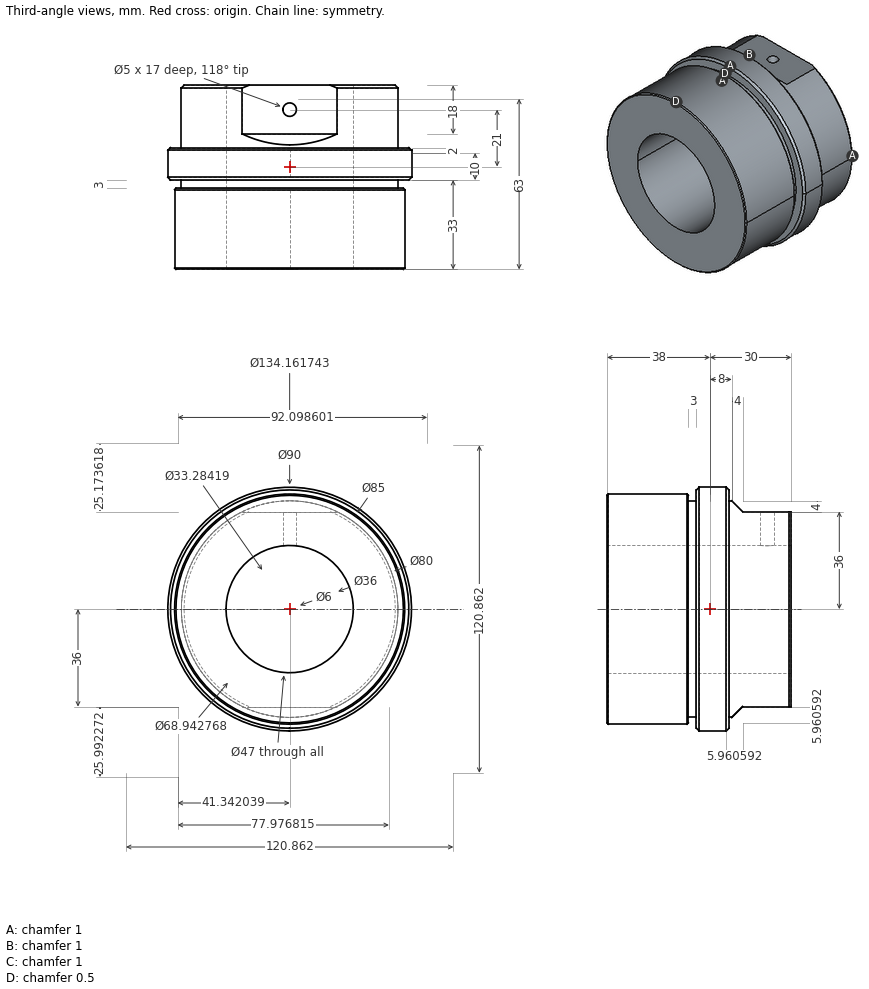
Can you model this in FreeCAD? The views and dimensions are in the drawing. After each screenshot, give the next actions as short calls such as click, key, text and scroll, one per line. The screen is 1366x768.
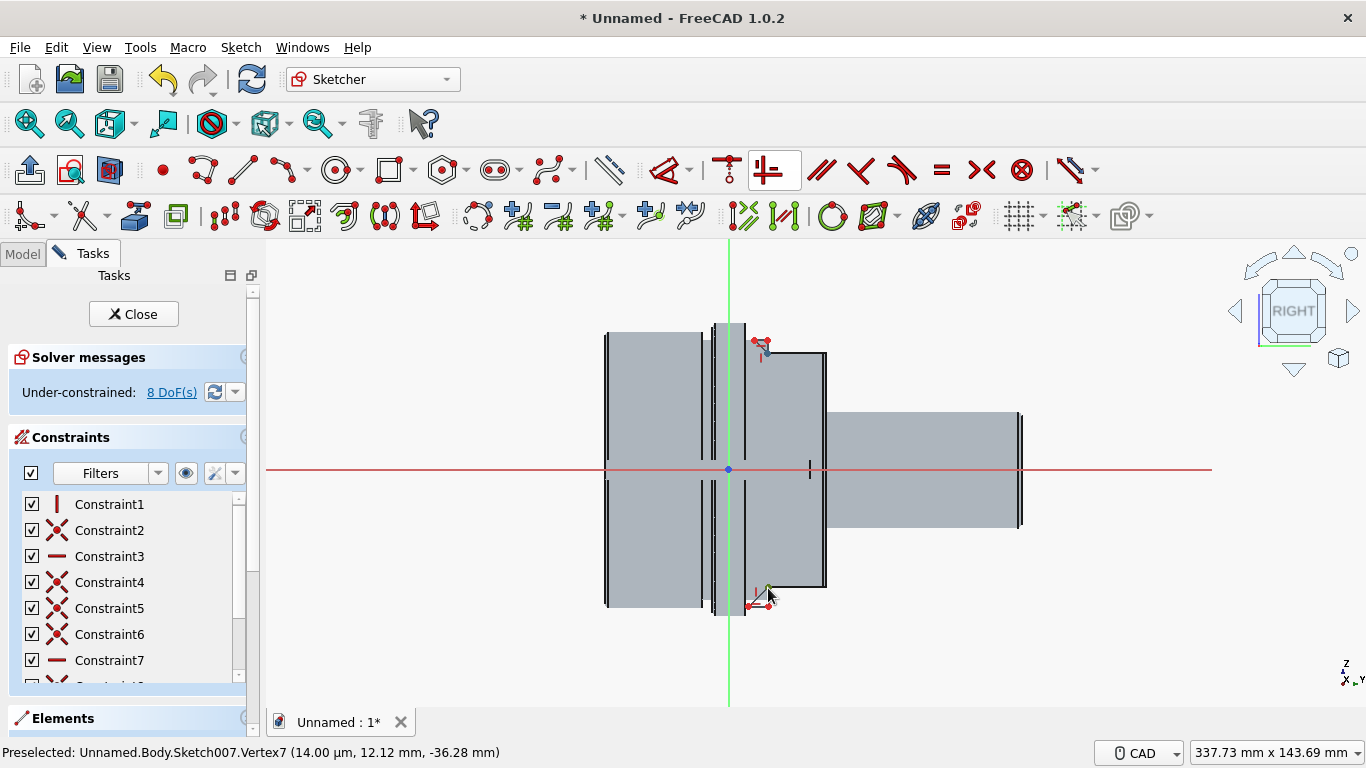
click(359, 470)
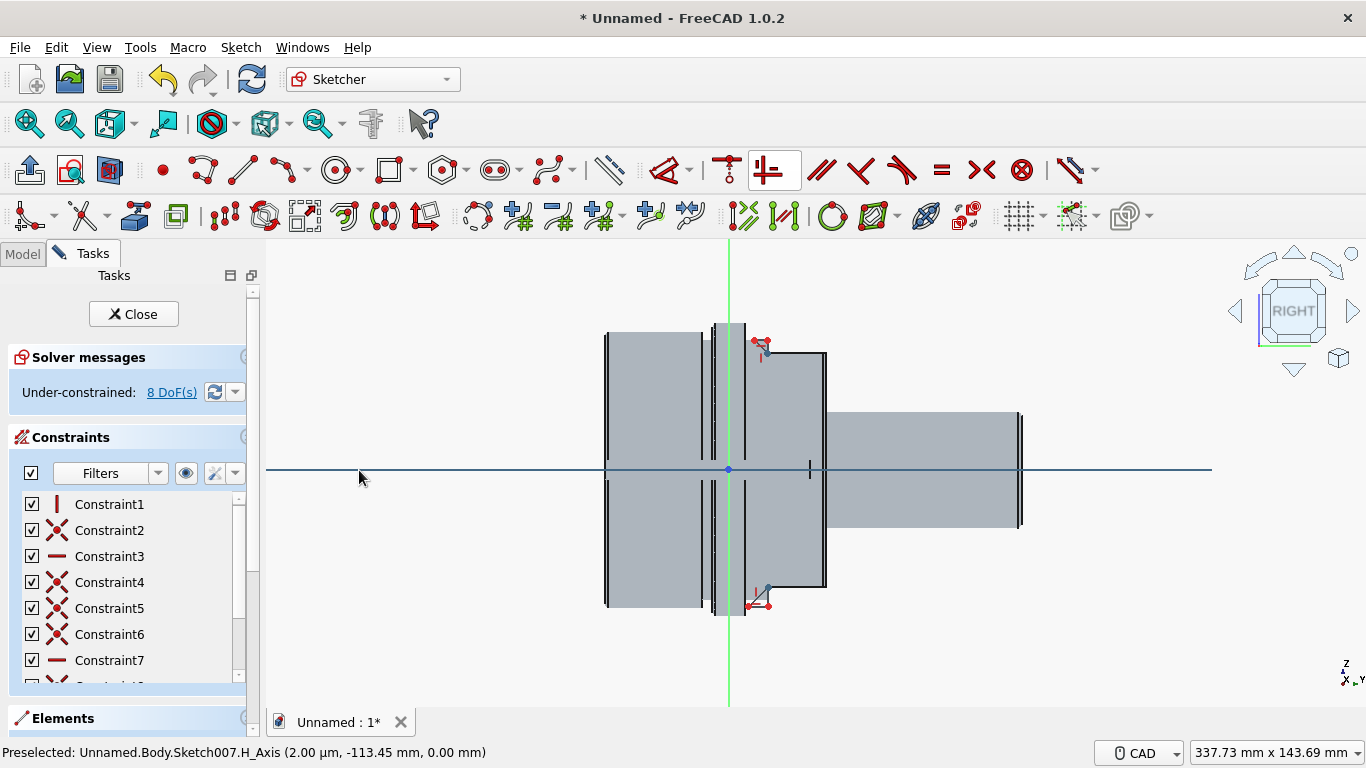
click(982, 170)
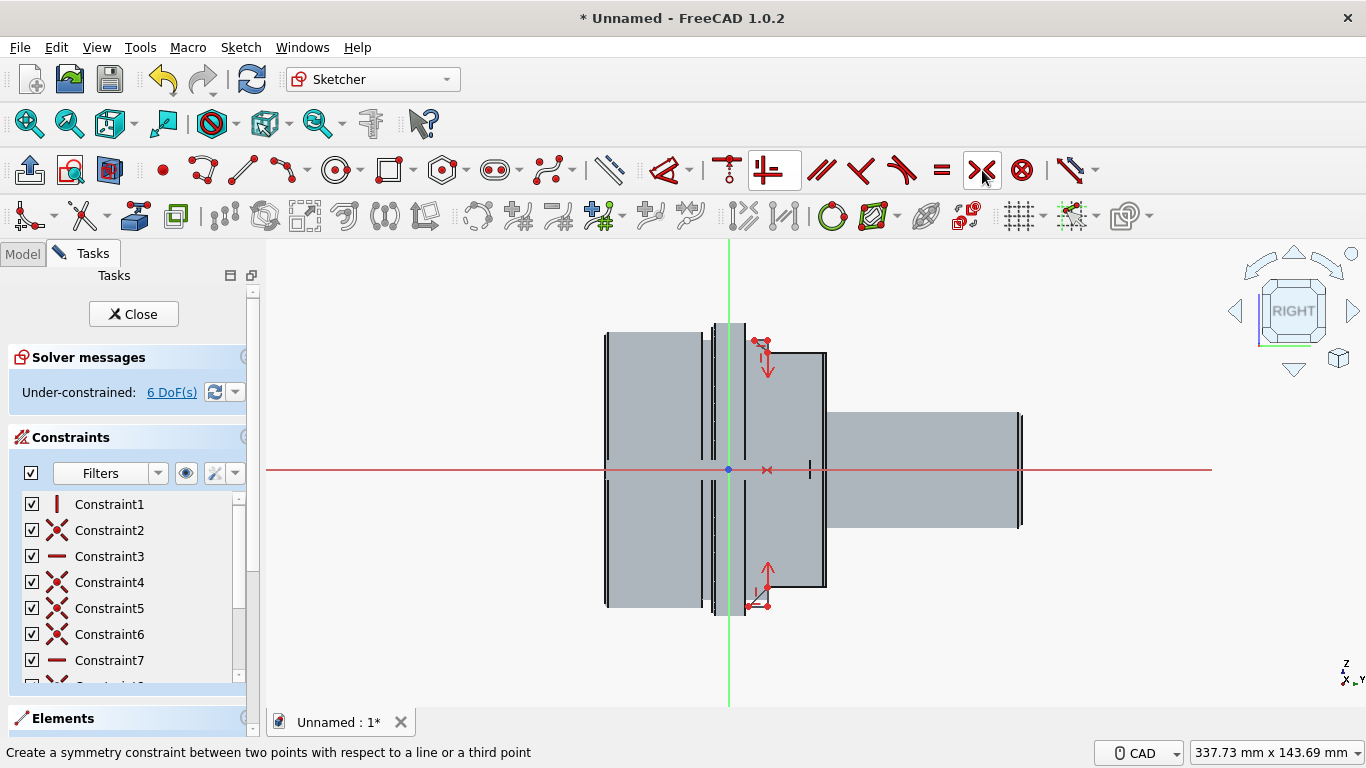
click(664, 170)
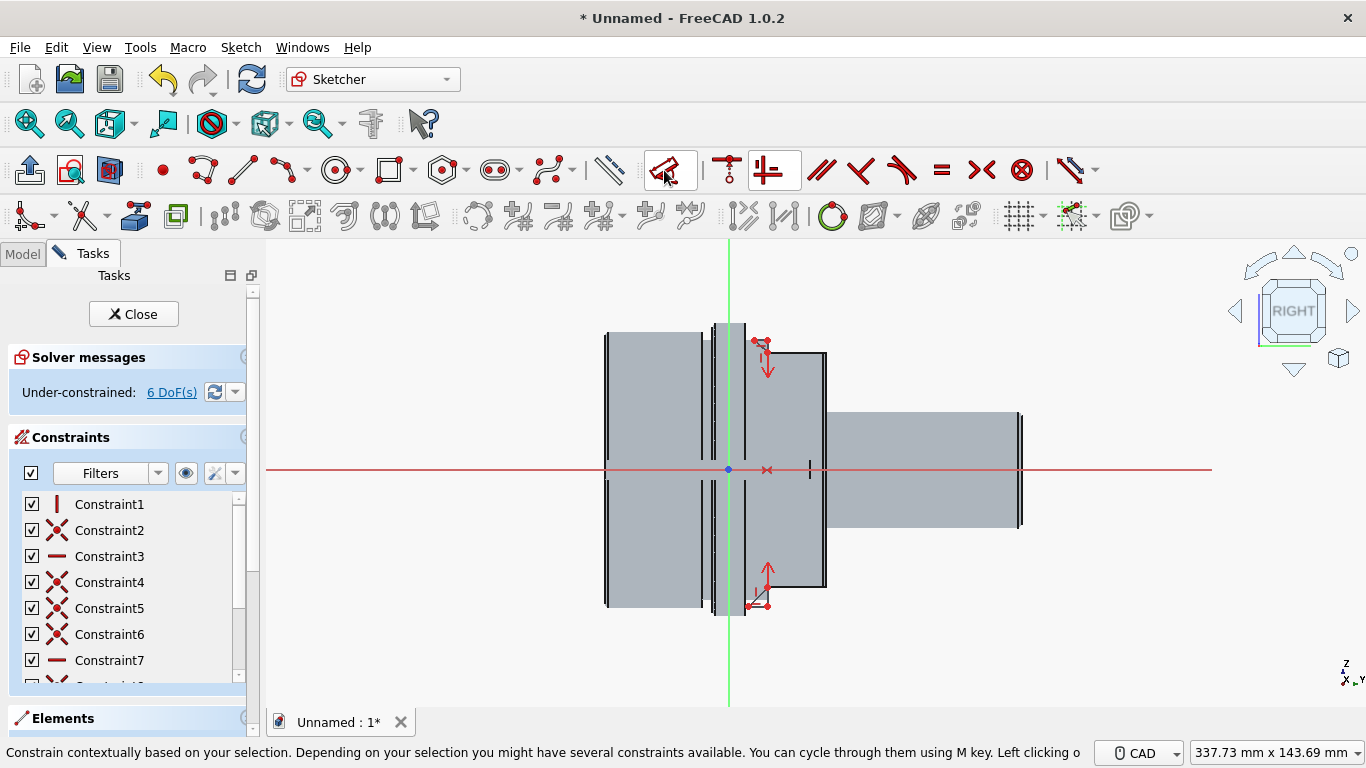
scroll(768, 345, up, 6)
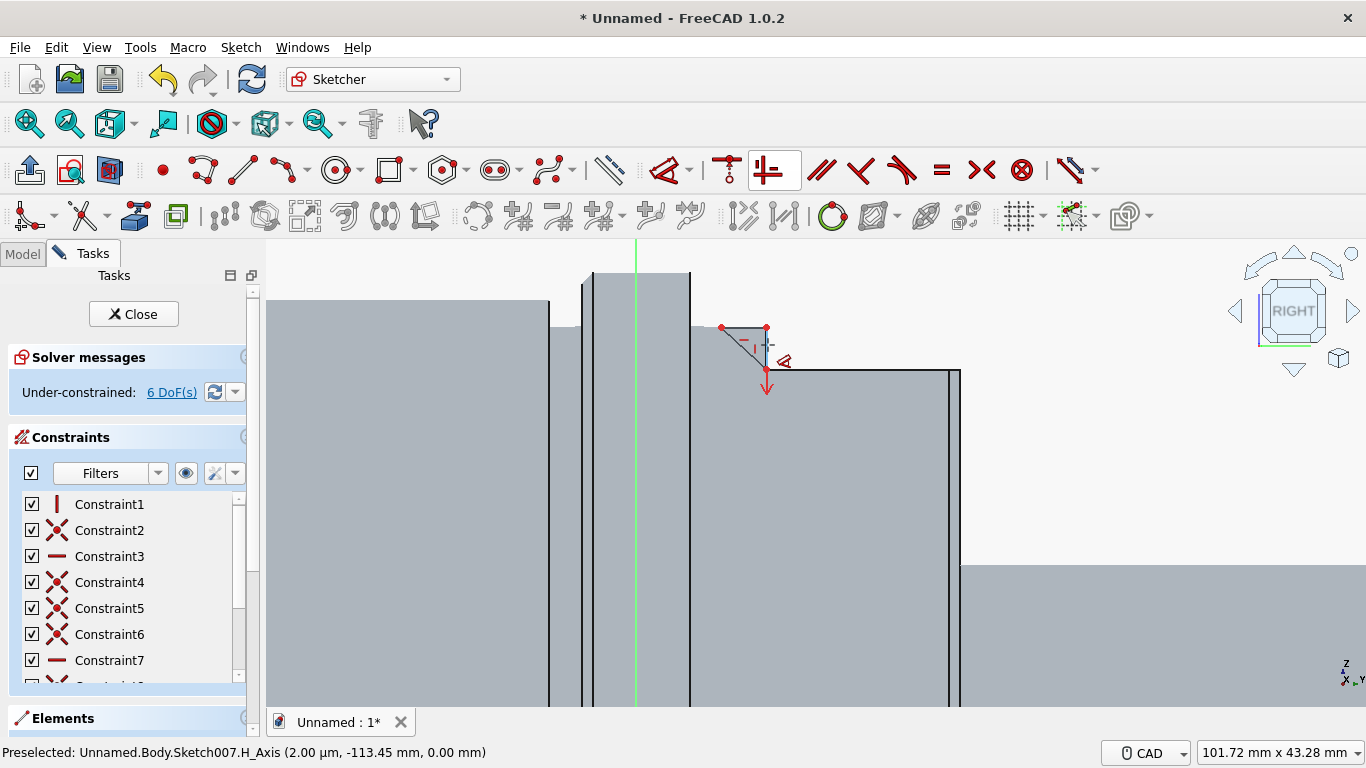
click(767, 345)
click(801, 349)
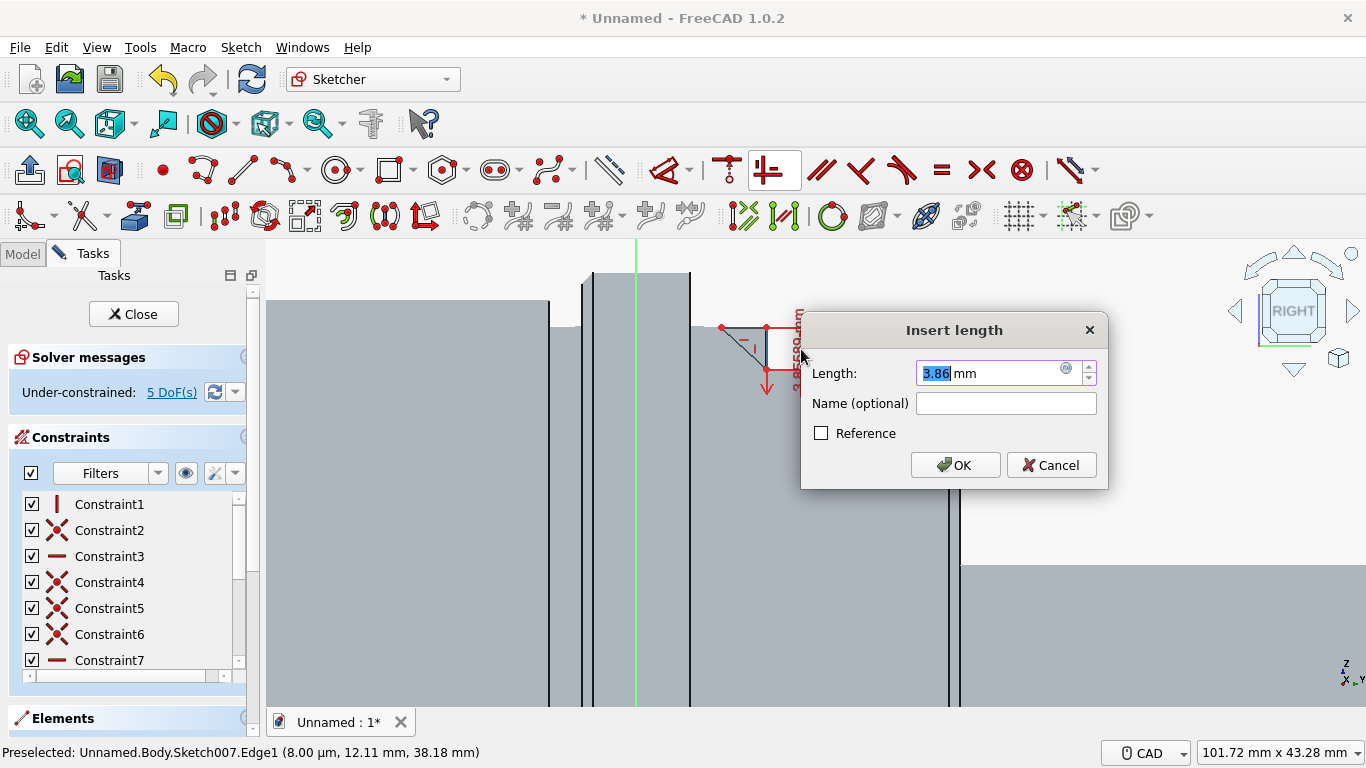
text(4)
key(Return)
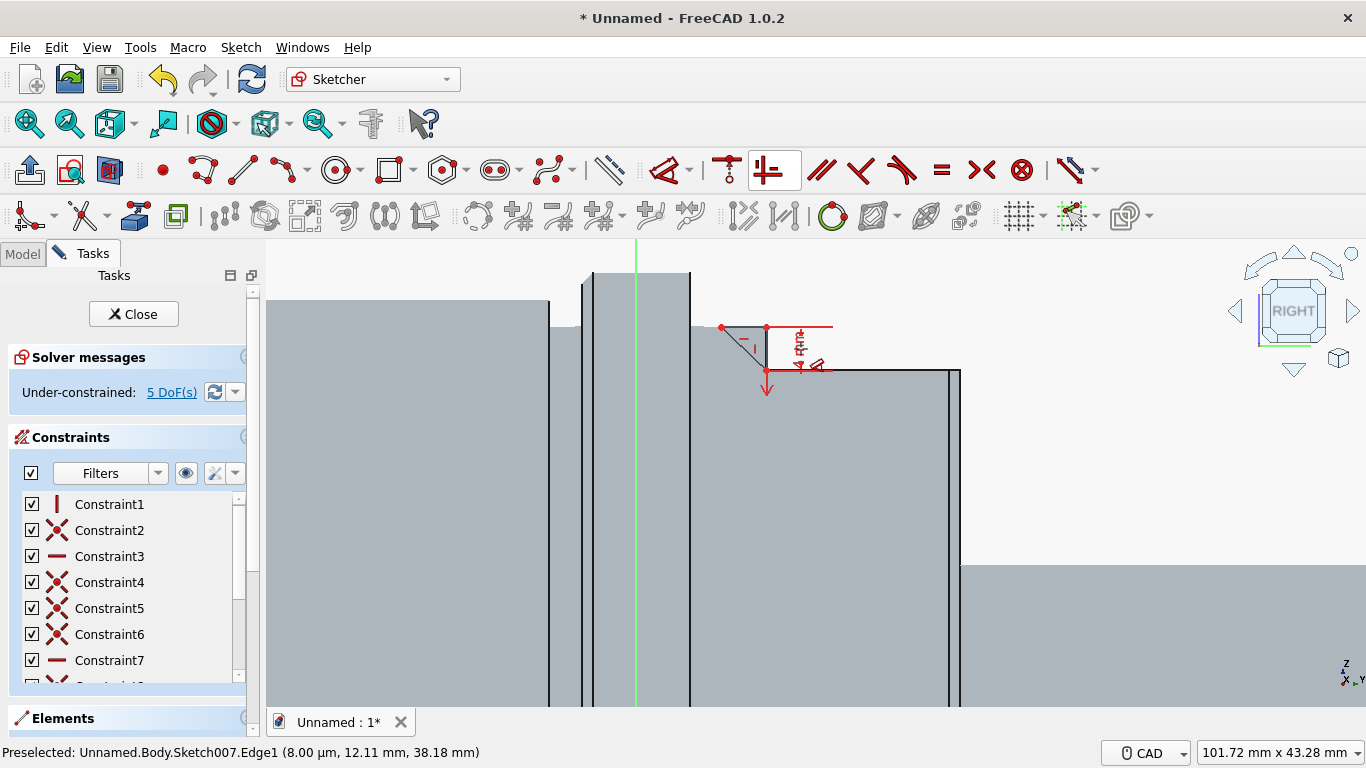
click(753, 327)
click(744, 293)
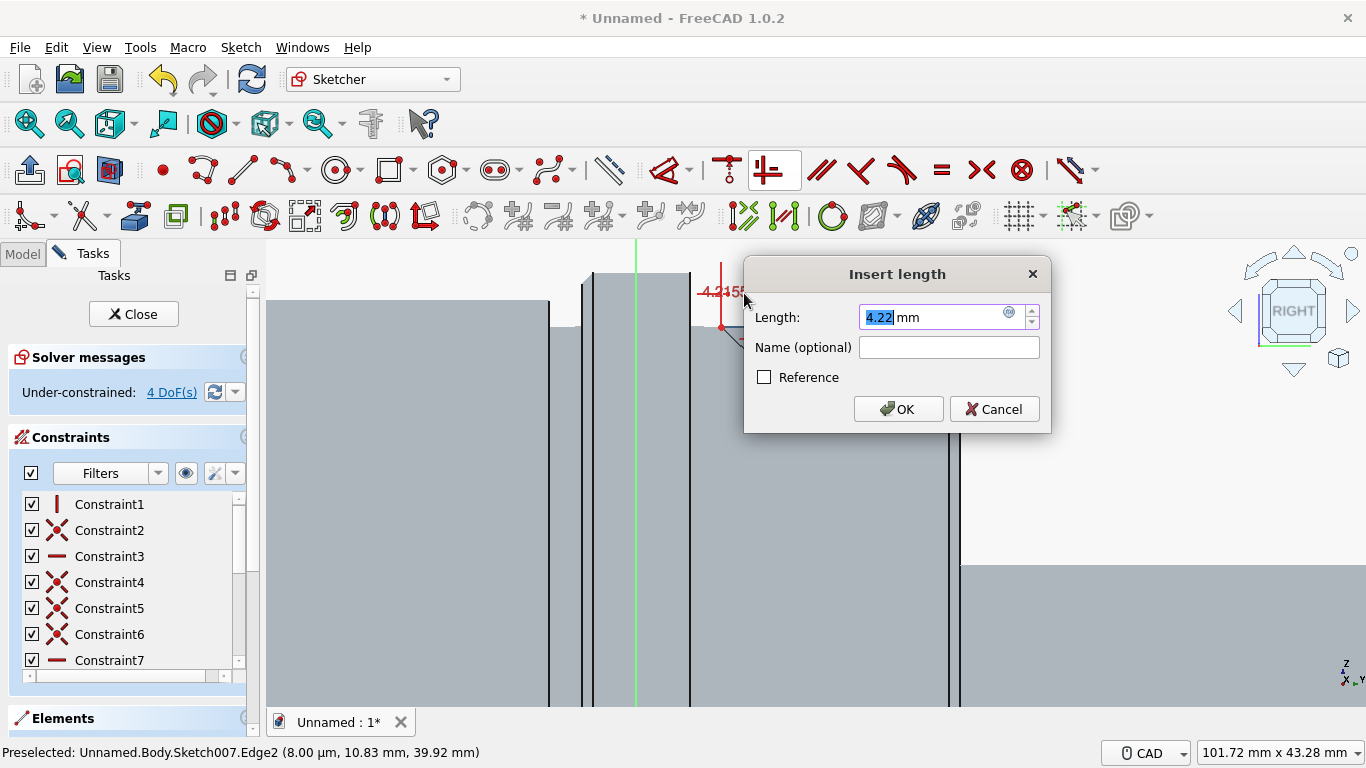
text(4)
key(Return)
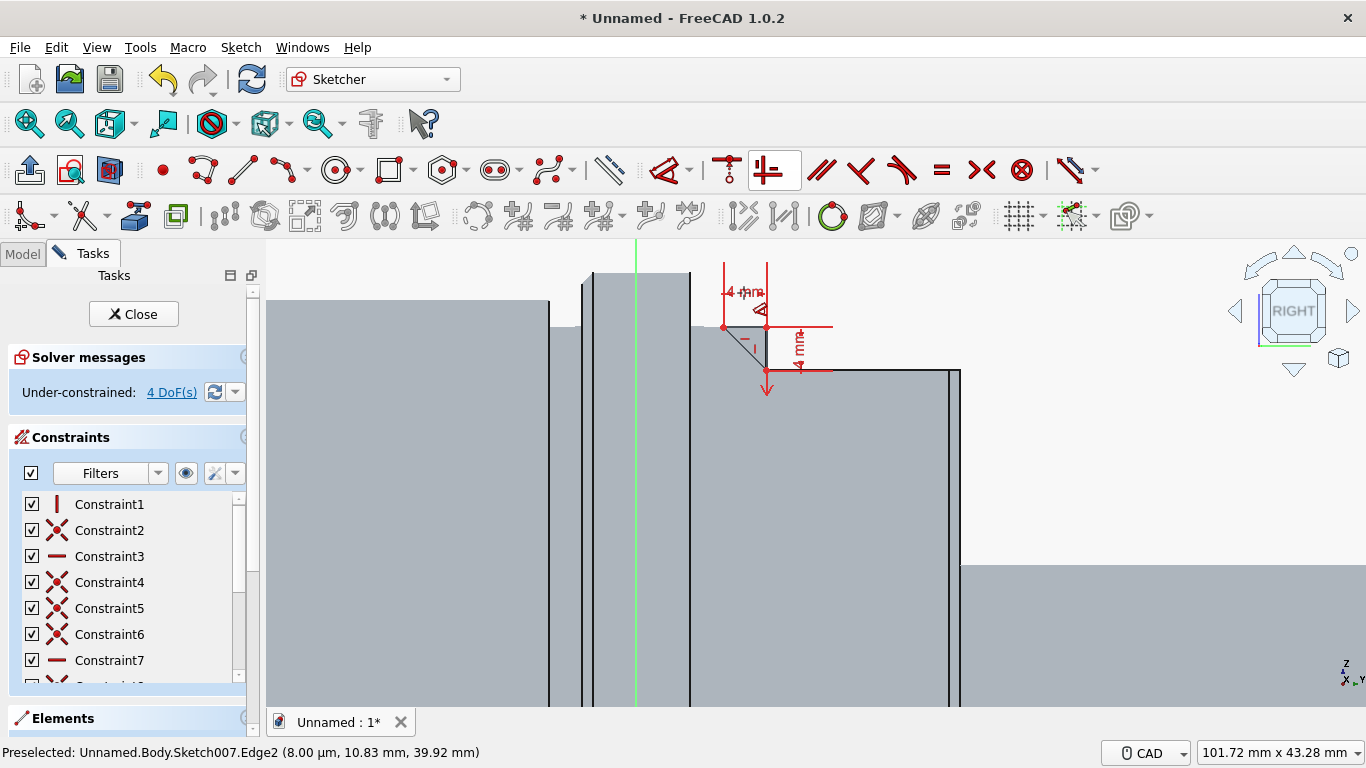
click(724, 327)
click(660, 293)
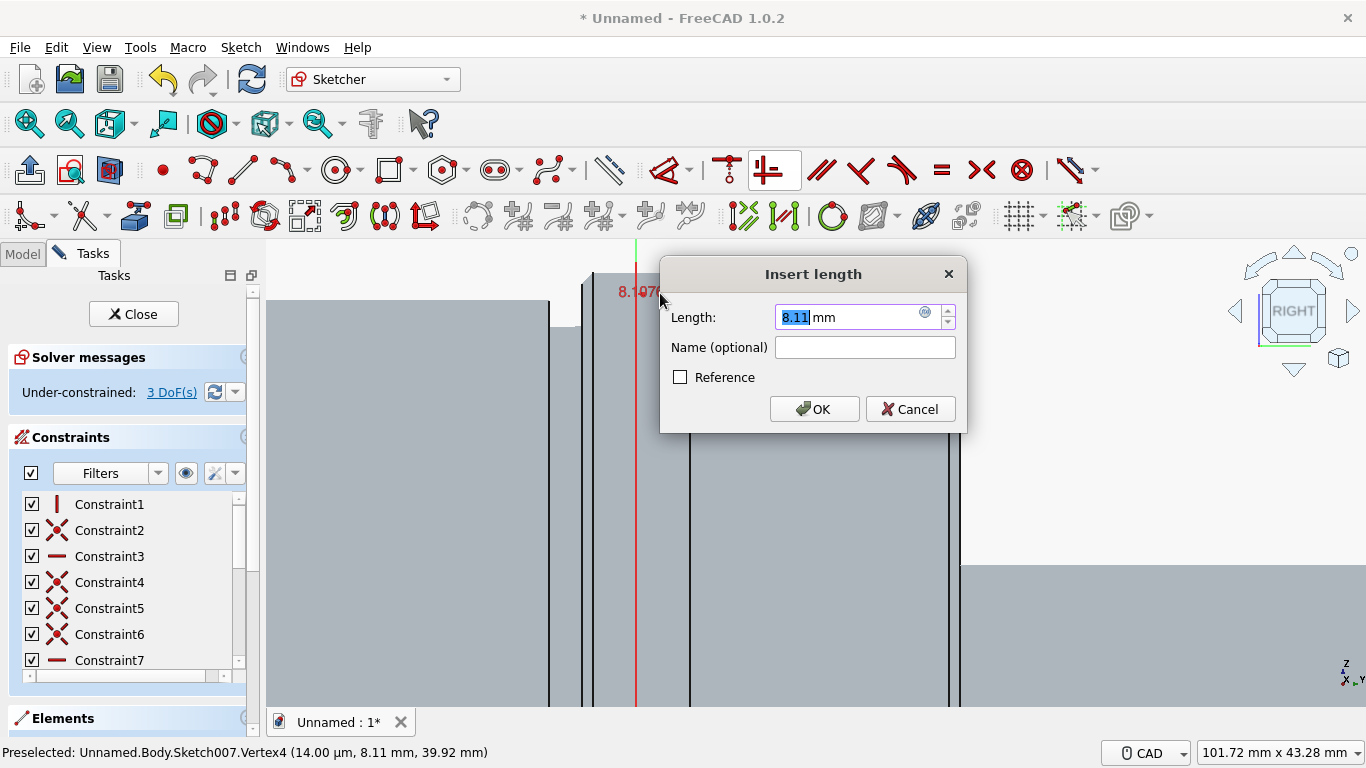
text(8)
key(Return)